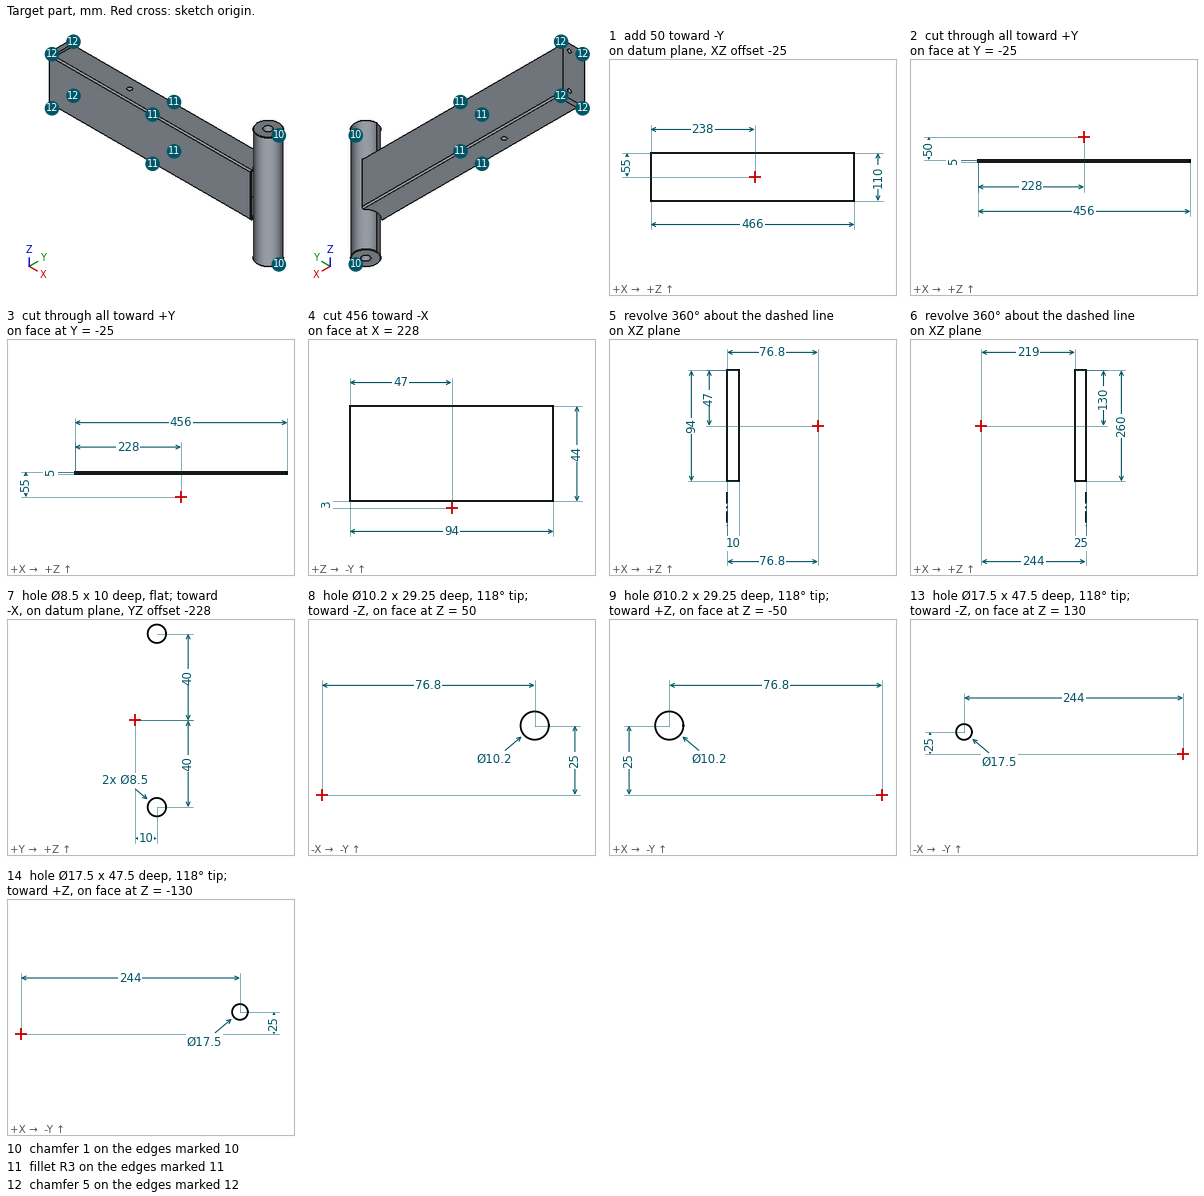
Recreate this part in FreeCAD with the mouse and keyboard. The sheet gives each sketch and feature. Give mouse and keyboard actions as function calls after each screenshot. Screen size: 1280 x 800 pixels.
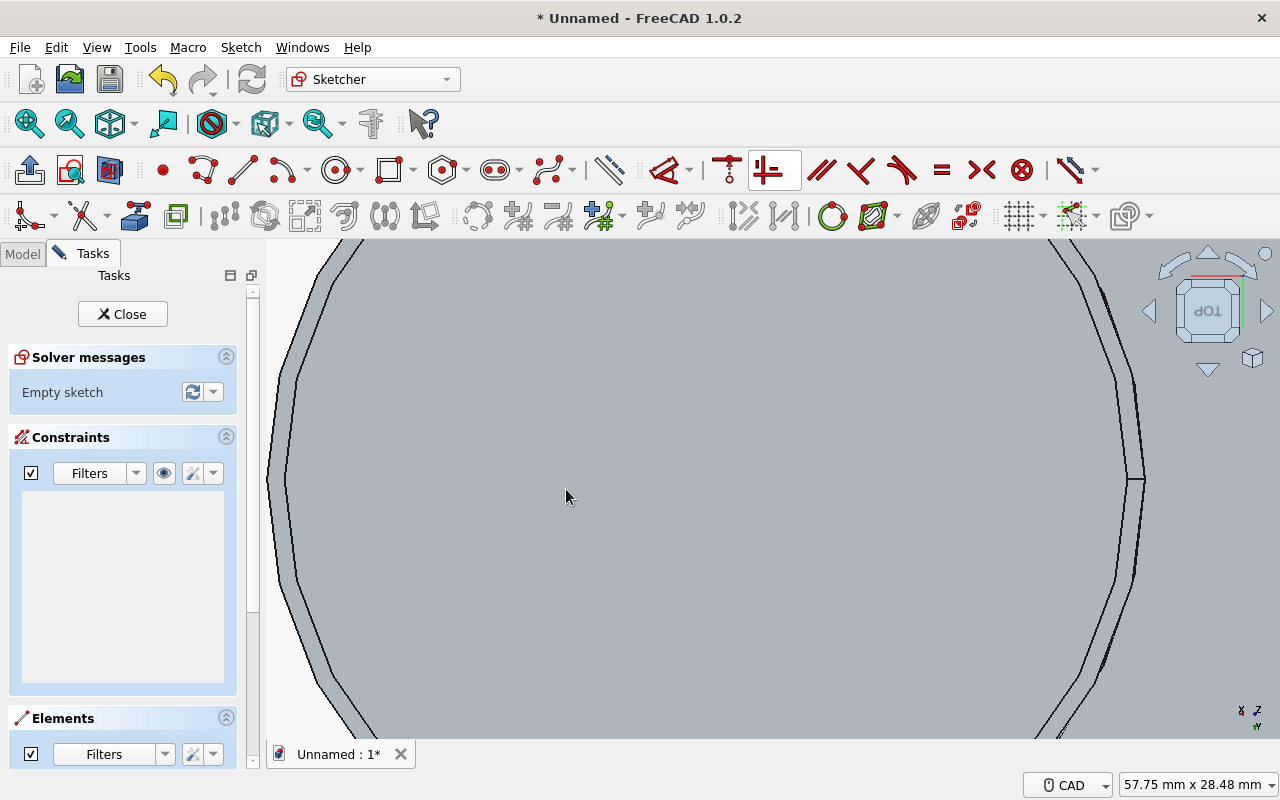
click(336, 170)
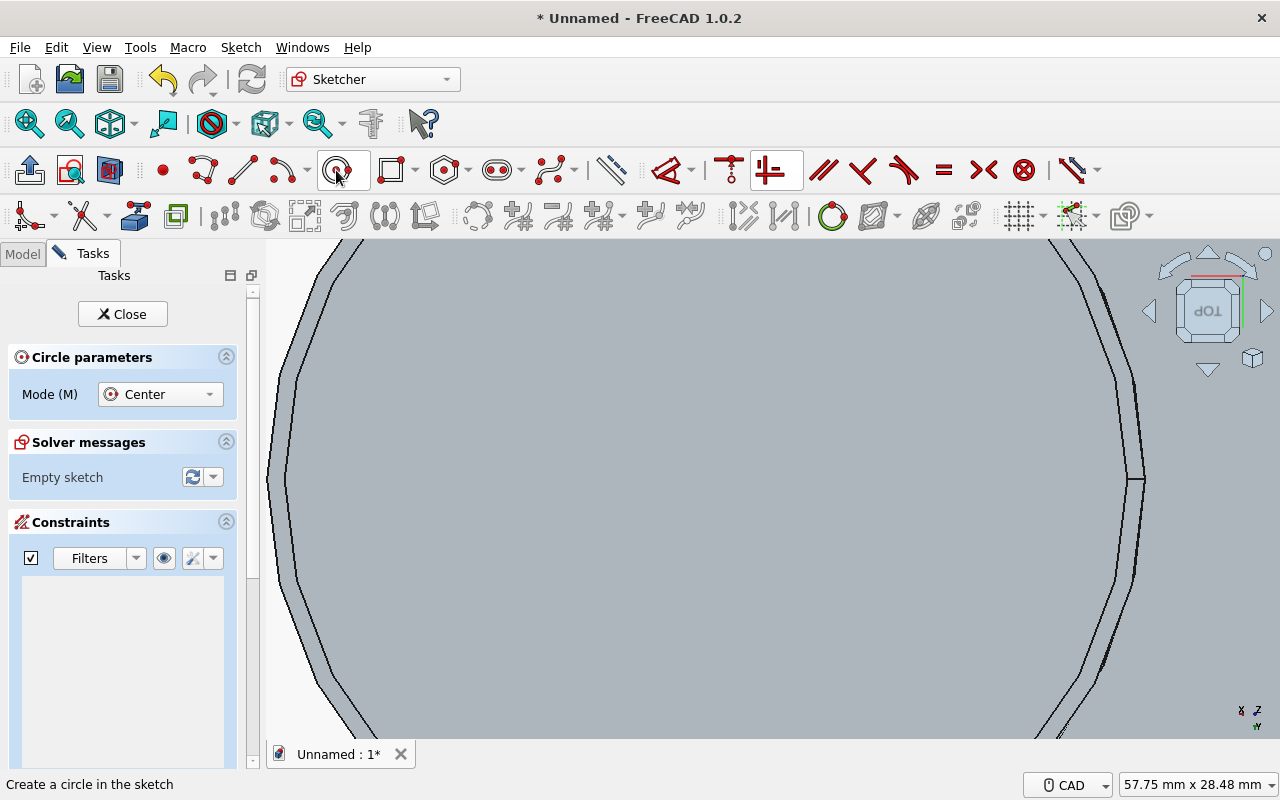
click(706, 479)
move(815, 371)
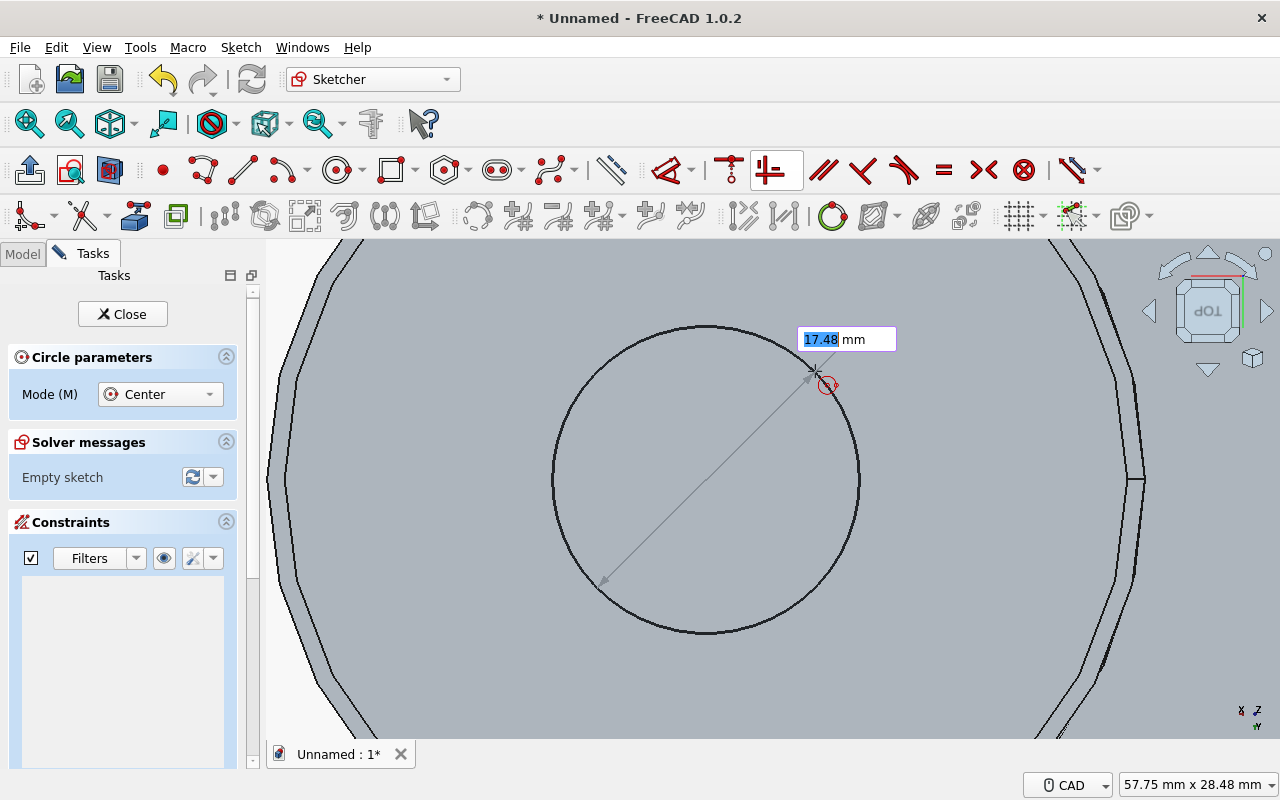
text(17.5)
key(Return)
key(Escape)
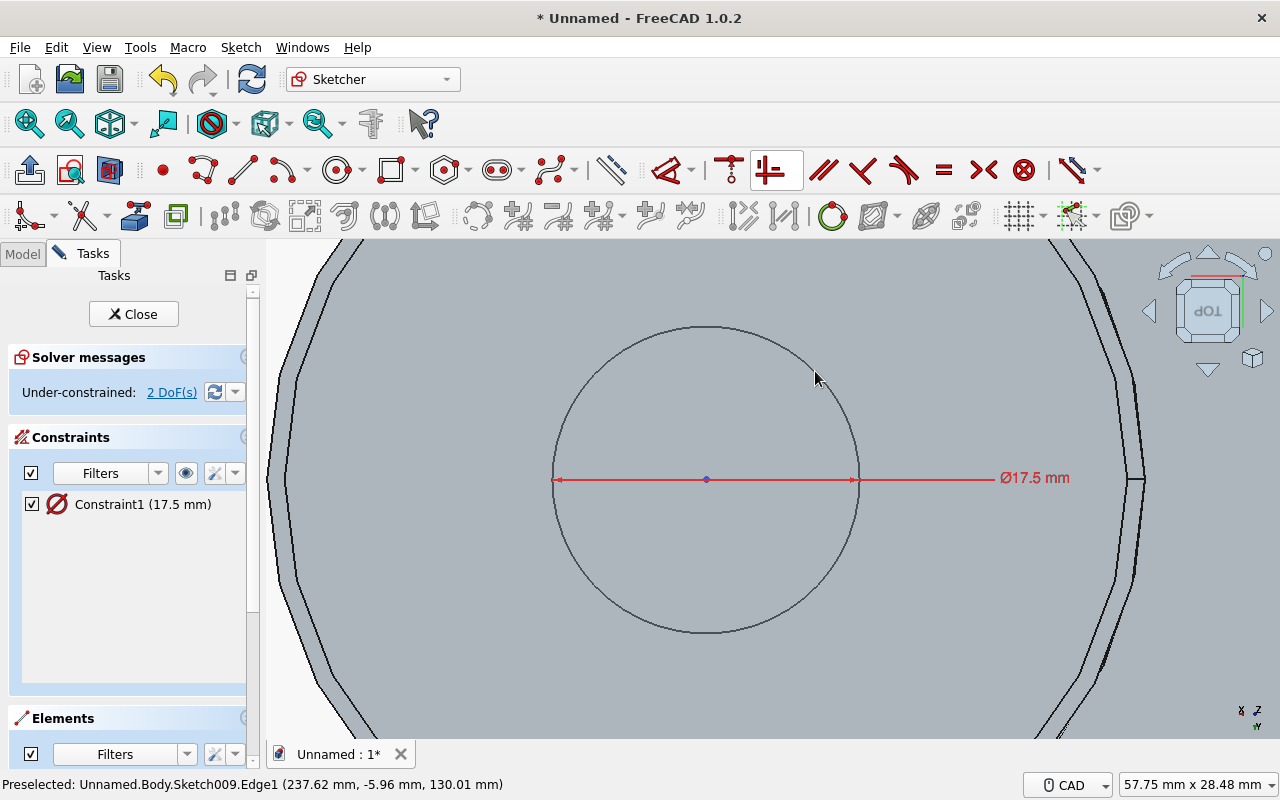
click(666, 170)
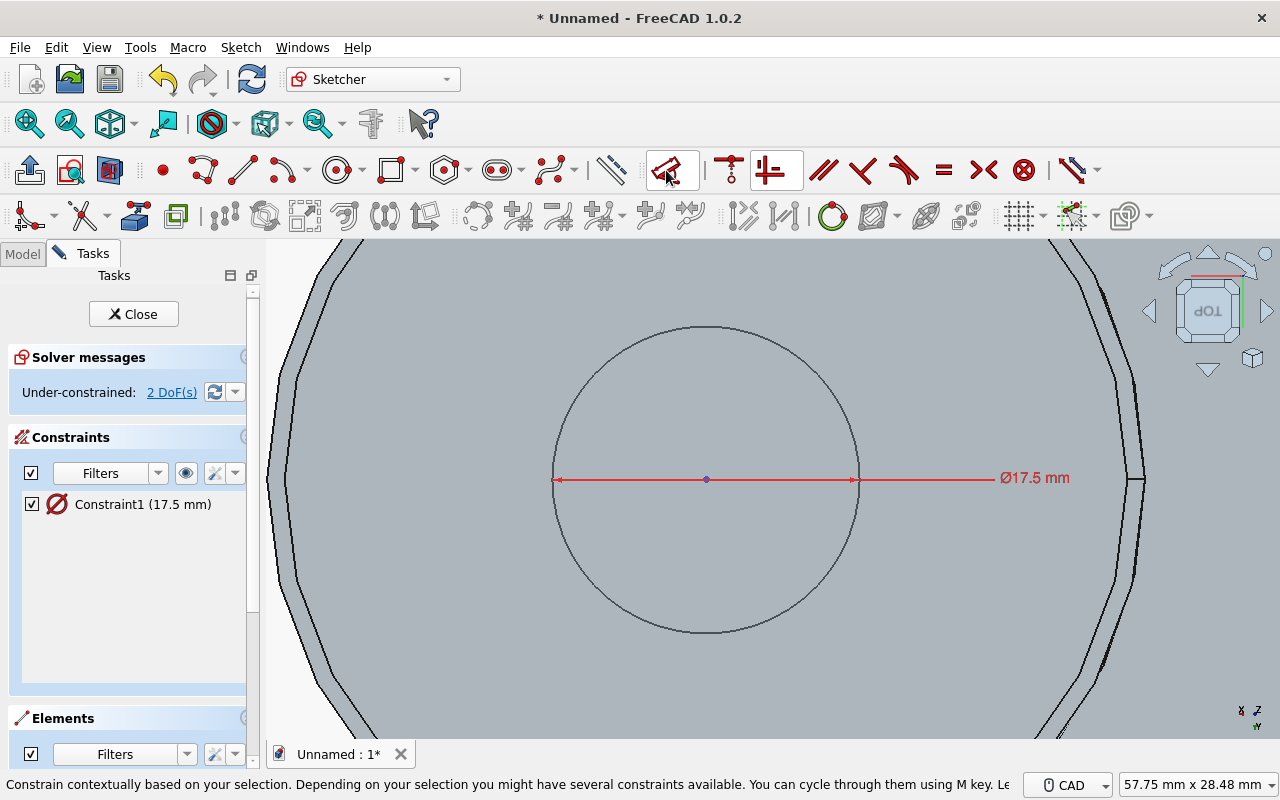
click(706, 480)
click(672, 596)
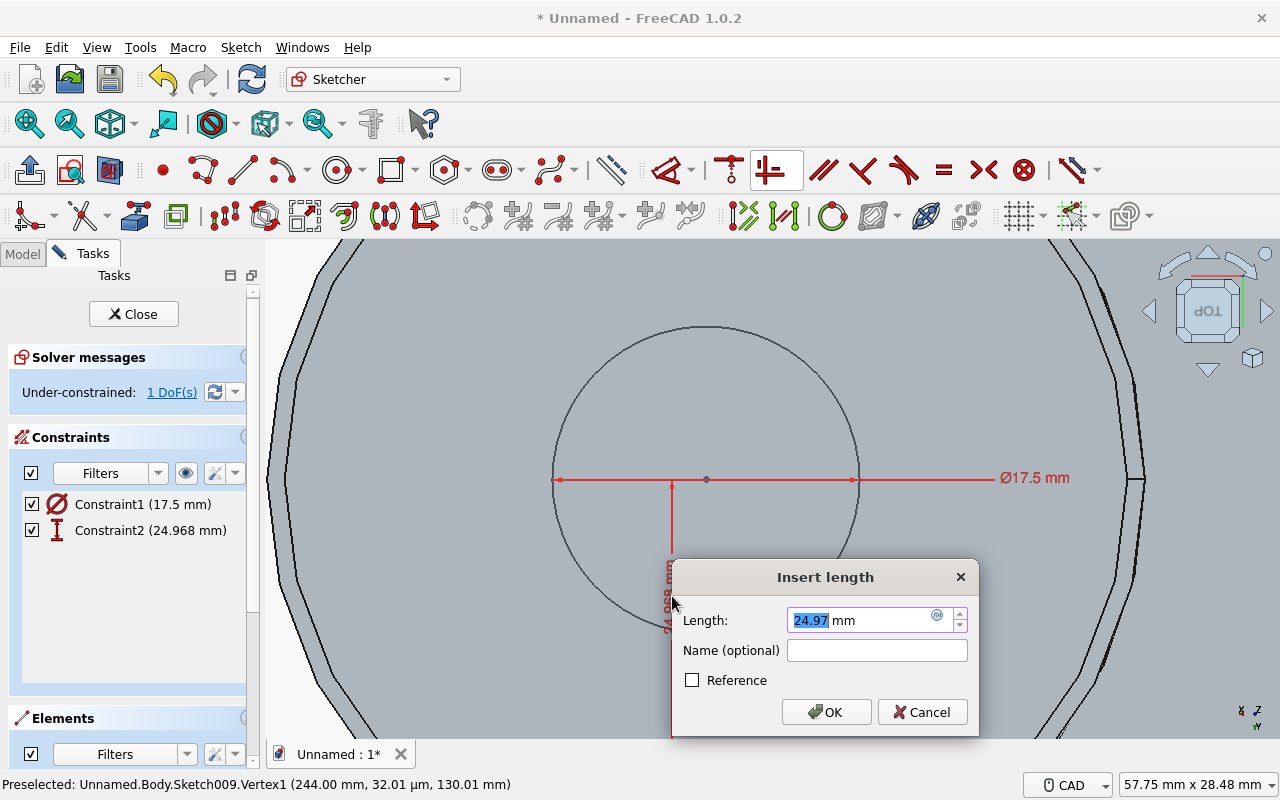
text(25)
key(Return)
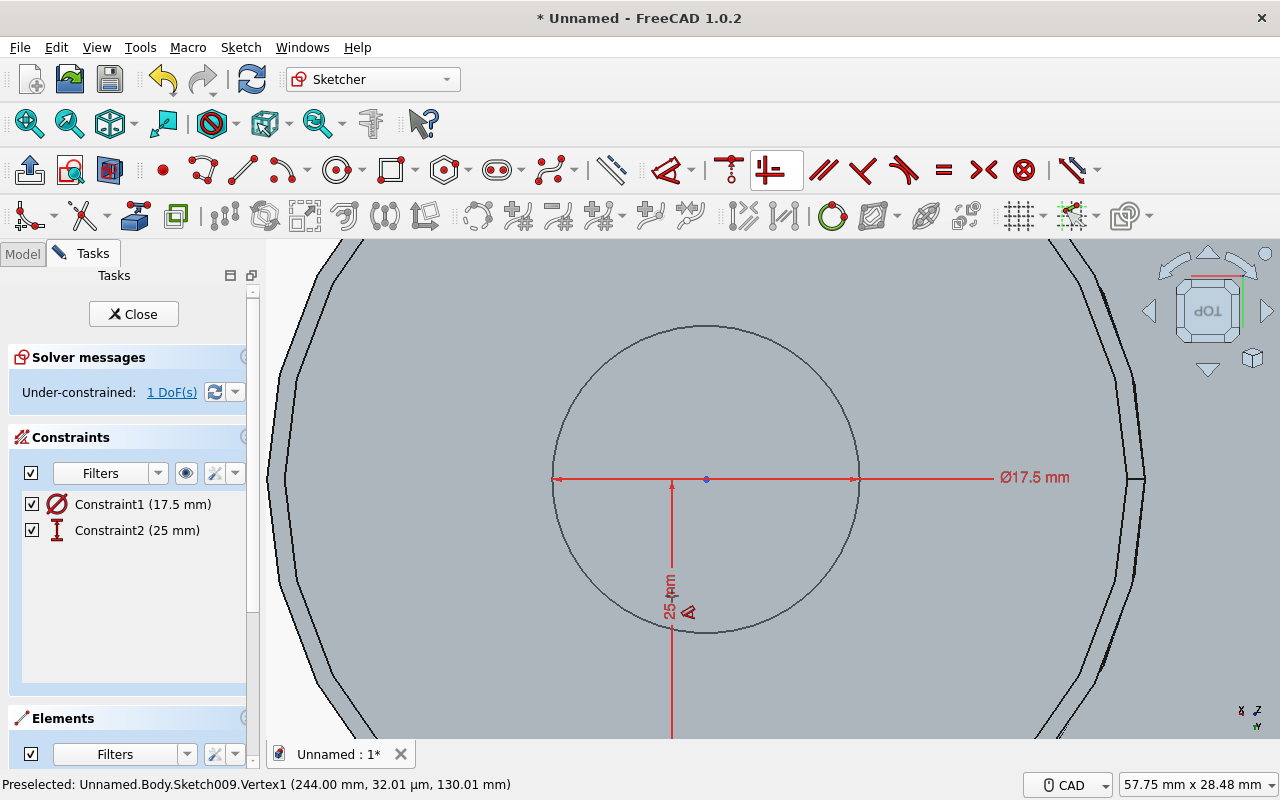
click(706, 479)
click(911, 445)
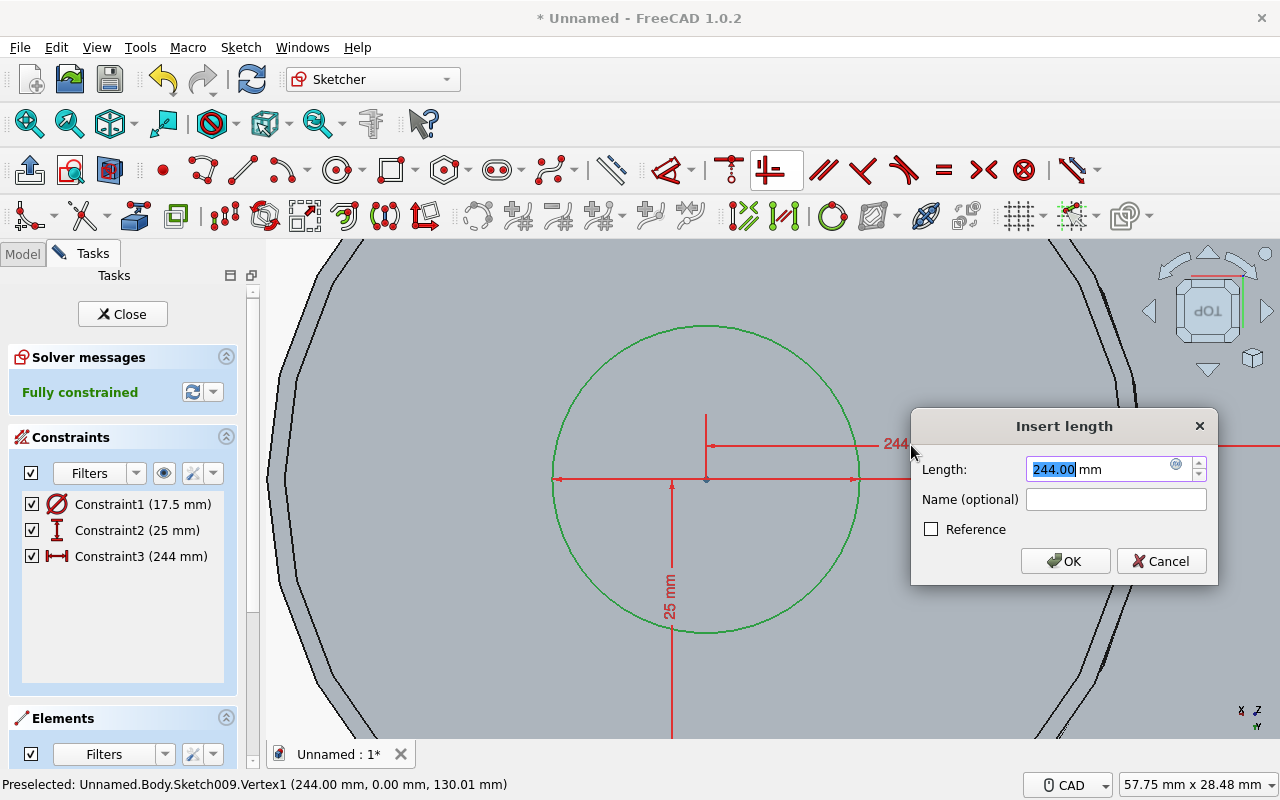
text(244)
key(Return)
key(Escape)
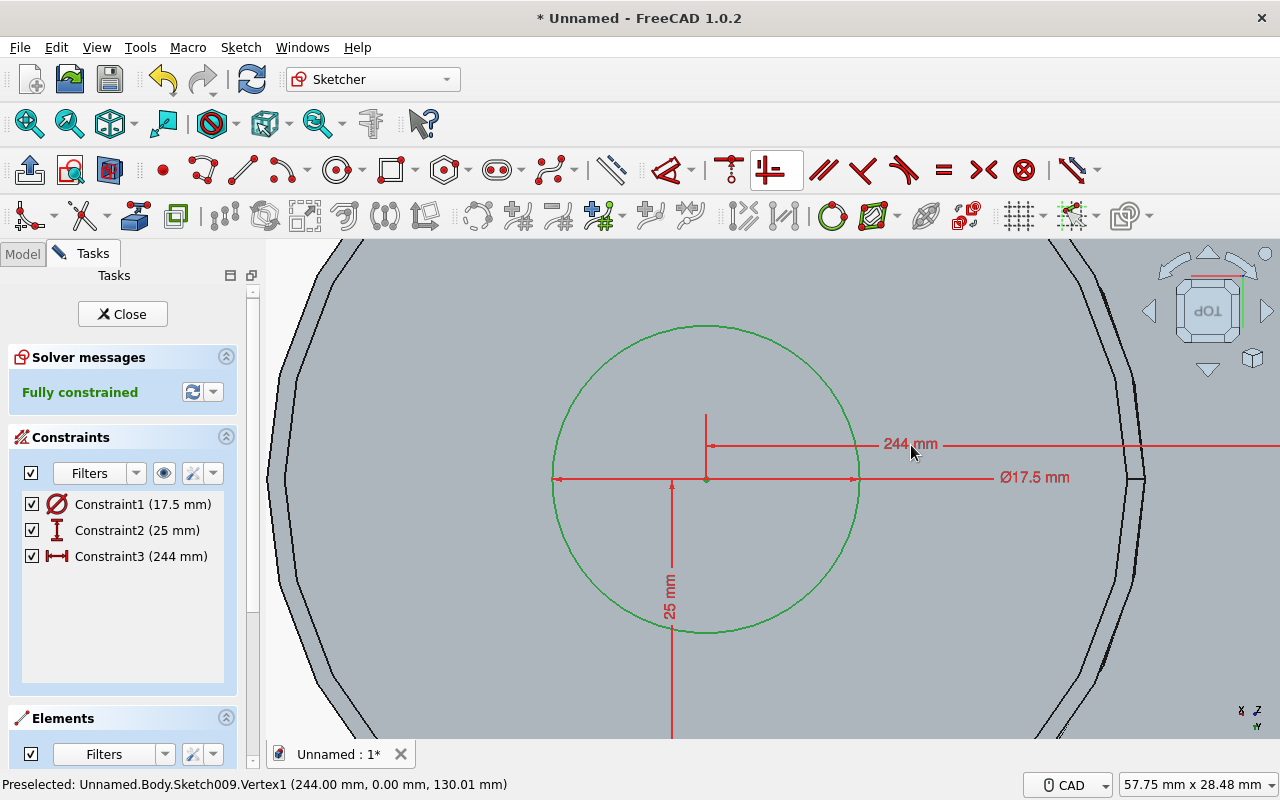
click(123, 314)